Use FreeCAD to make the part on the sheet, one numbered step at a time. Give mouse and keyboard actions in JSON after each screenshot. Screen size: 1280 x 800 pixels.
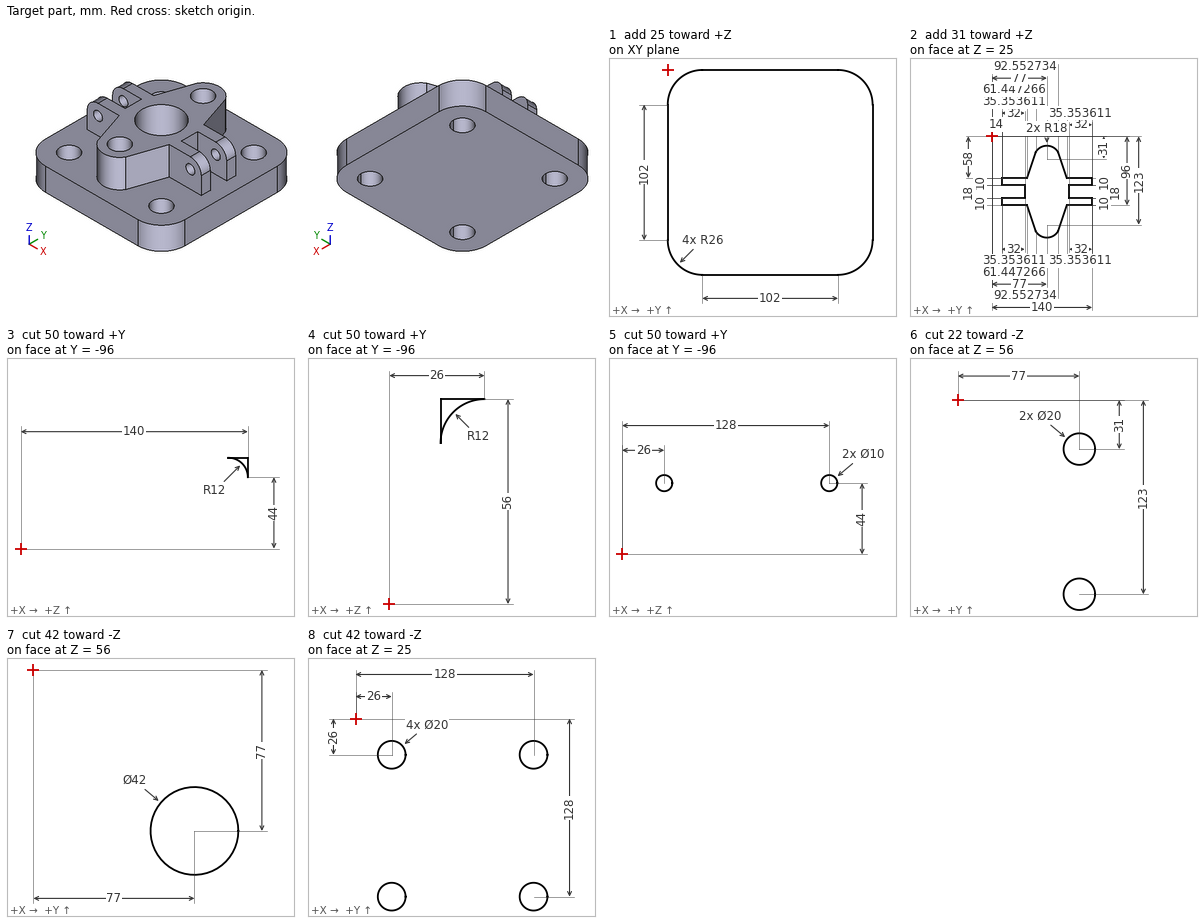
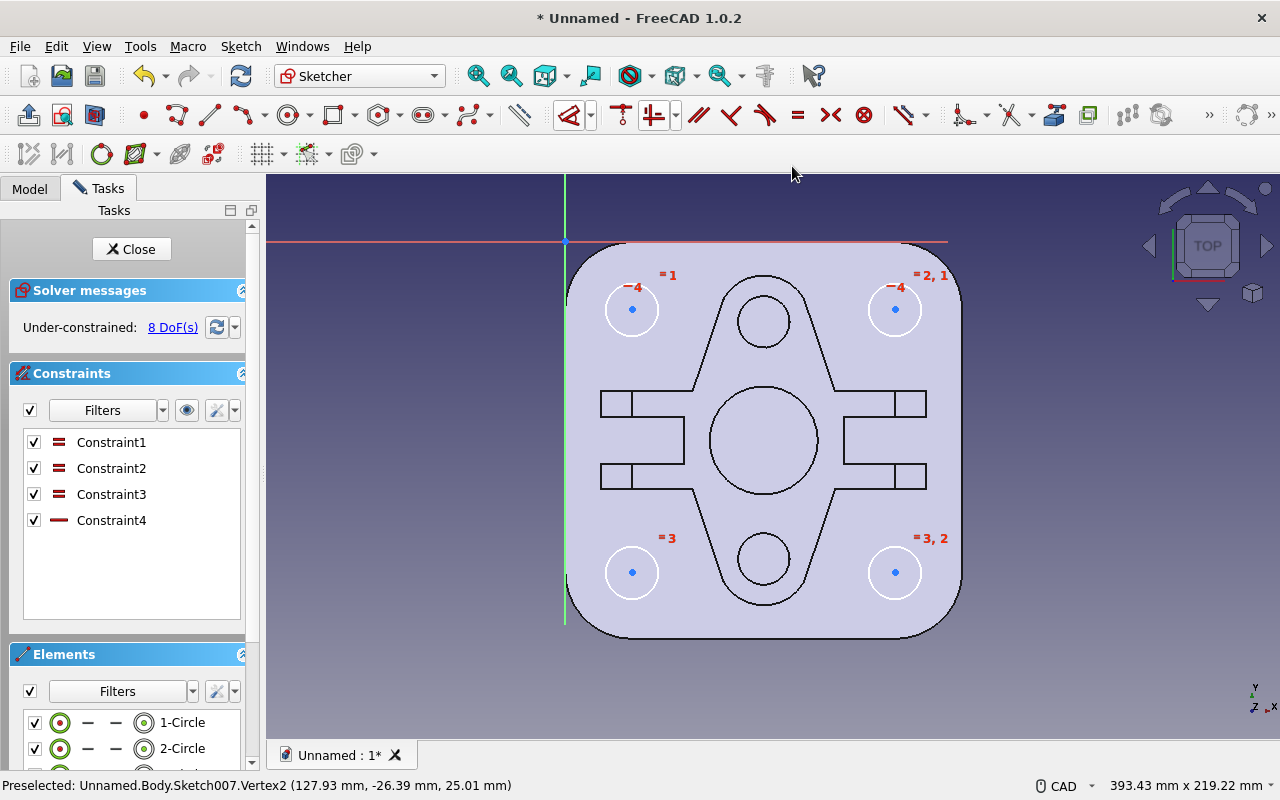
{"action": "left_click", "coordinate": [895, 310]}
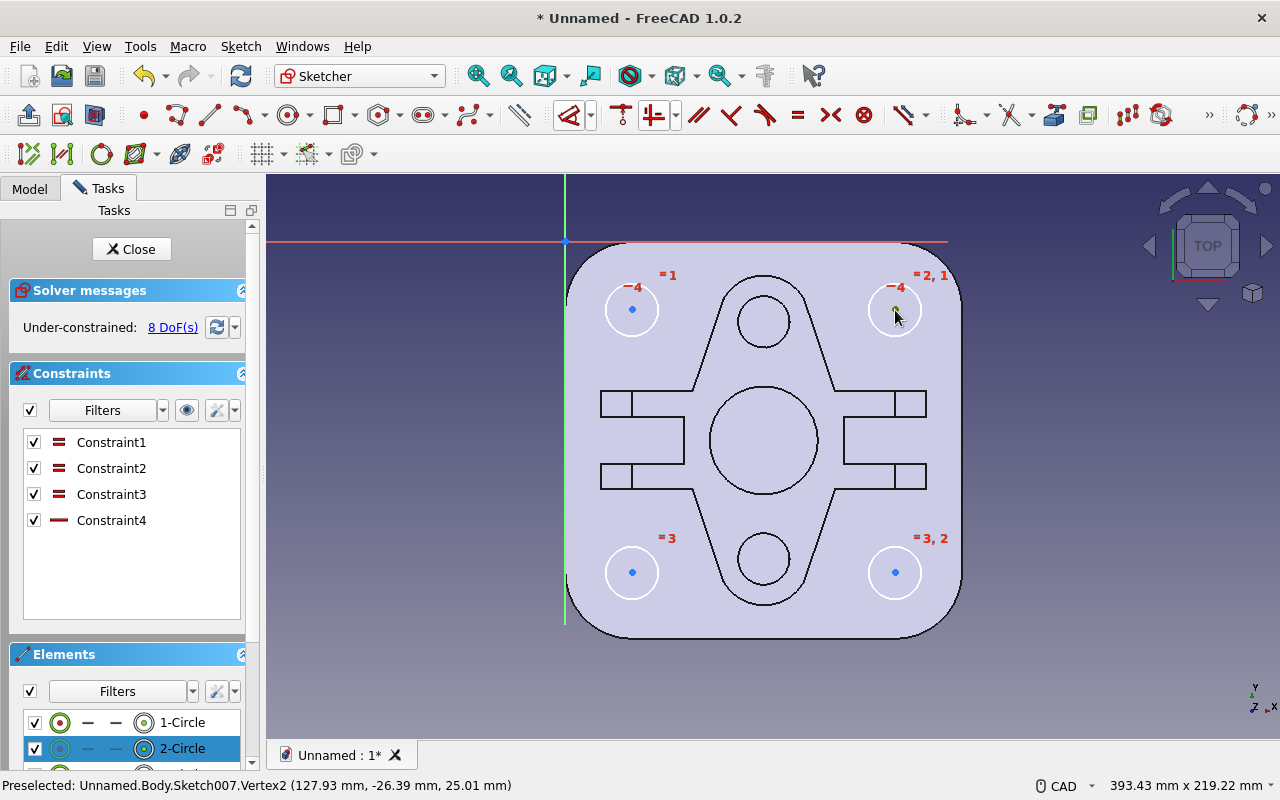
{"action": "left_click", "coordinate": [895, 573]}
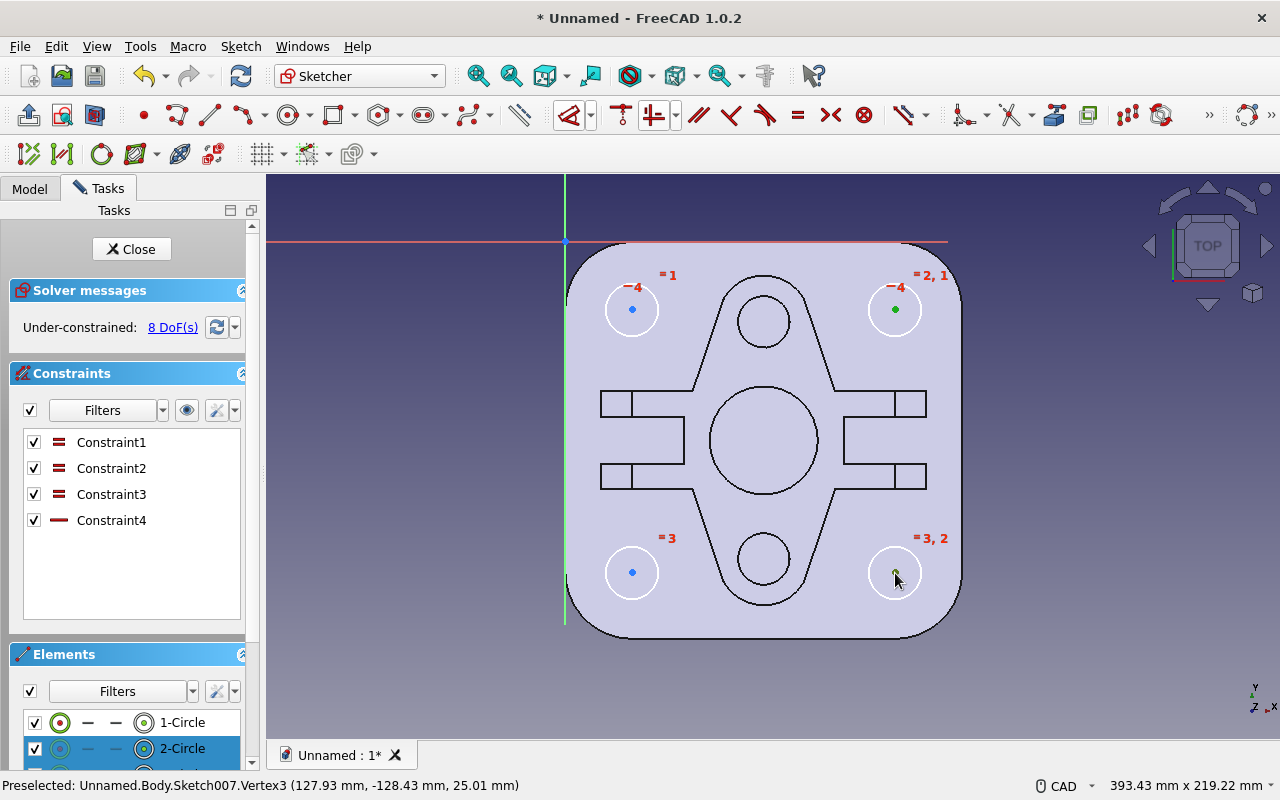
{"action": "key", "text": "v"}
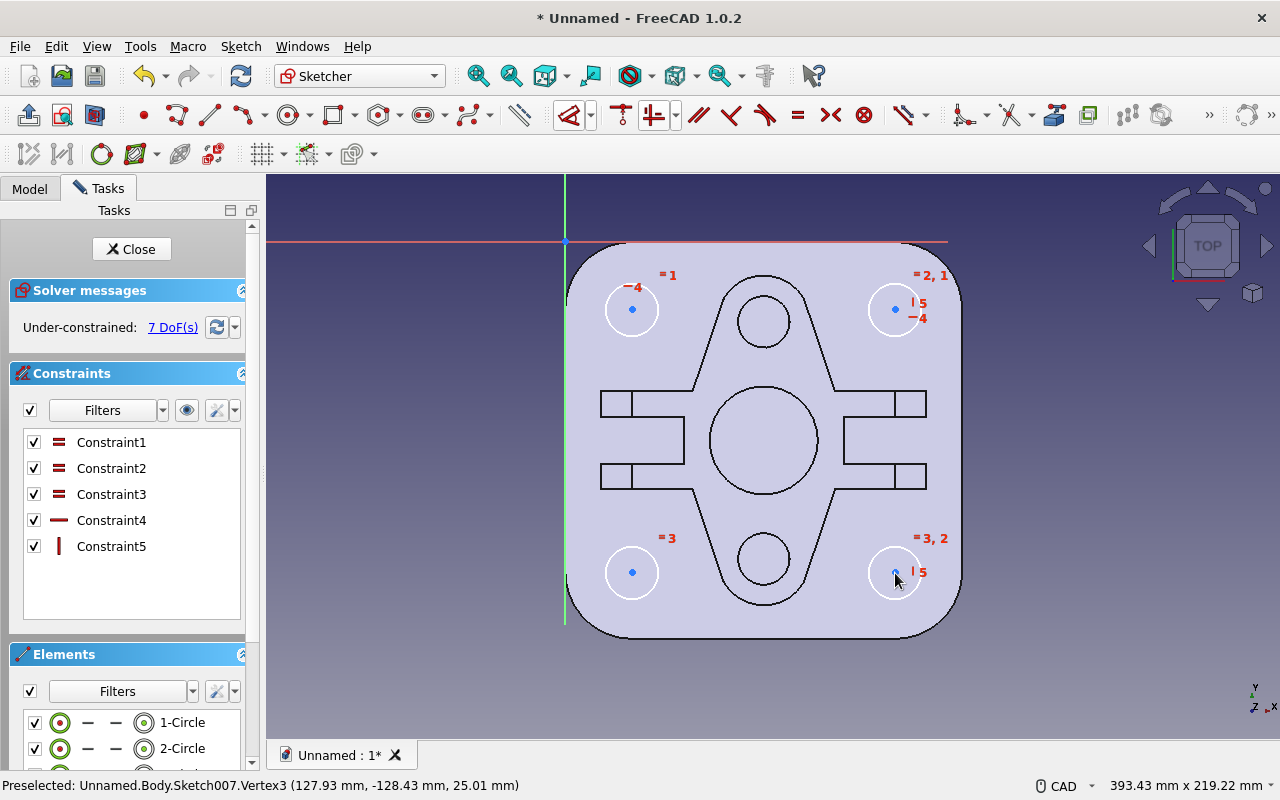
{"action": "left_click", "coordinate": [632, 310]}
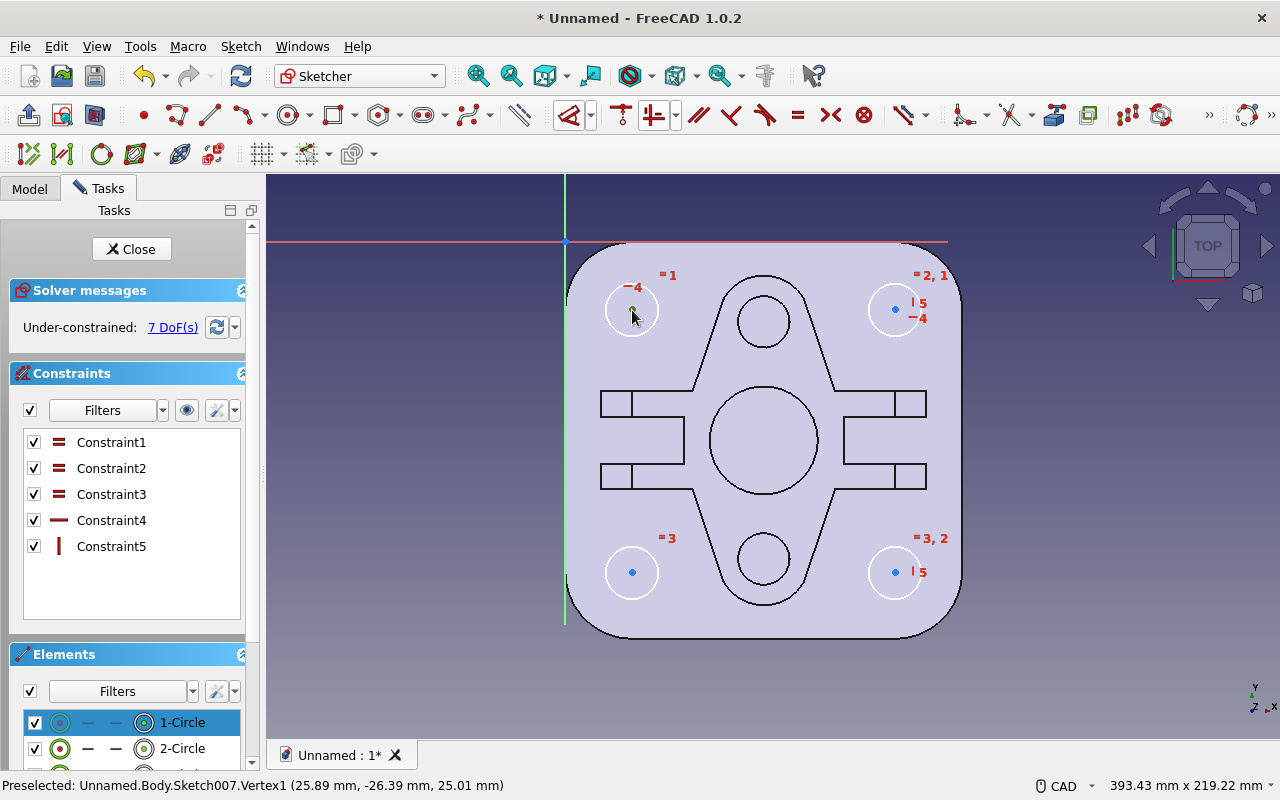
{"action": "left_click", "coordinate": [632, 573]}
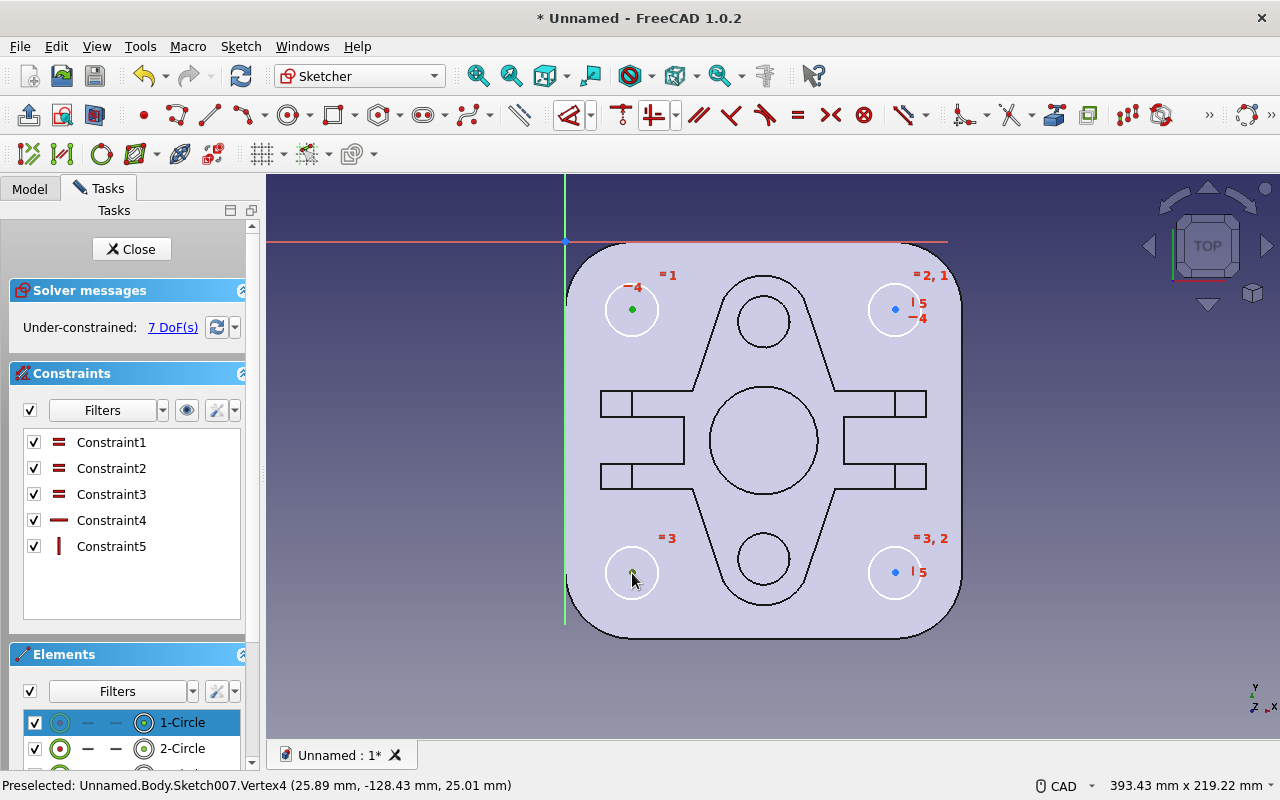
{"action": "left_click", "coordinate": [676, 116]}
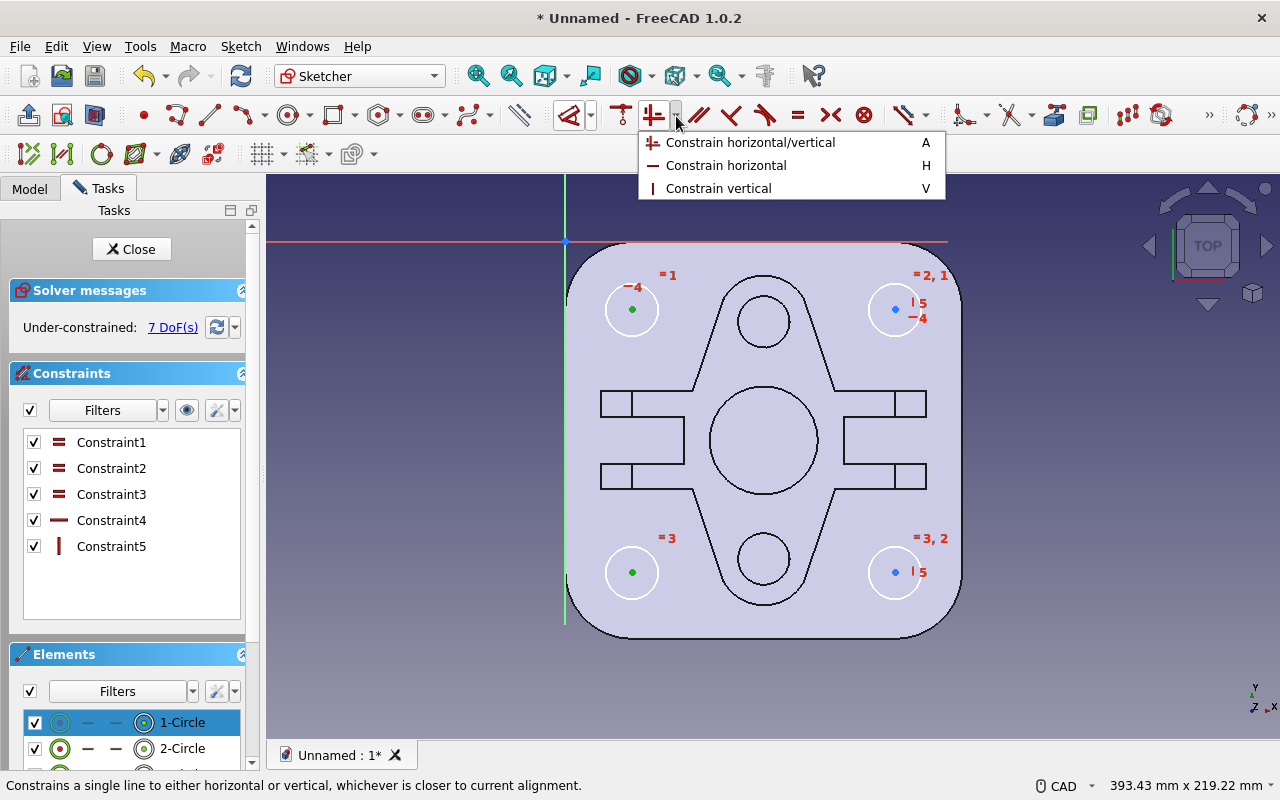
{"action": "left_click", "coordinate": [792, 188]}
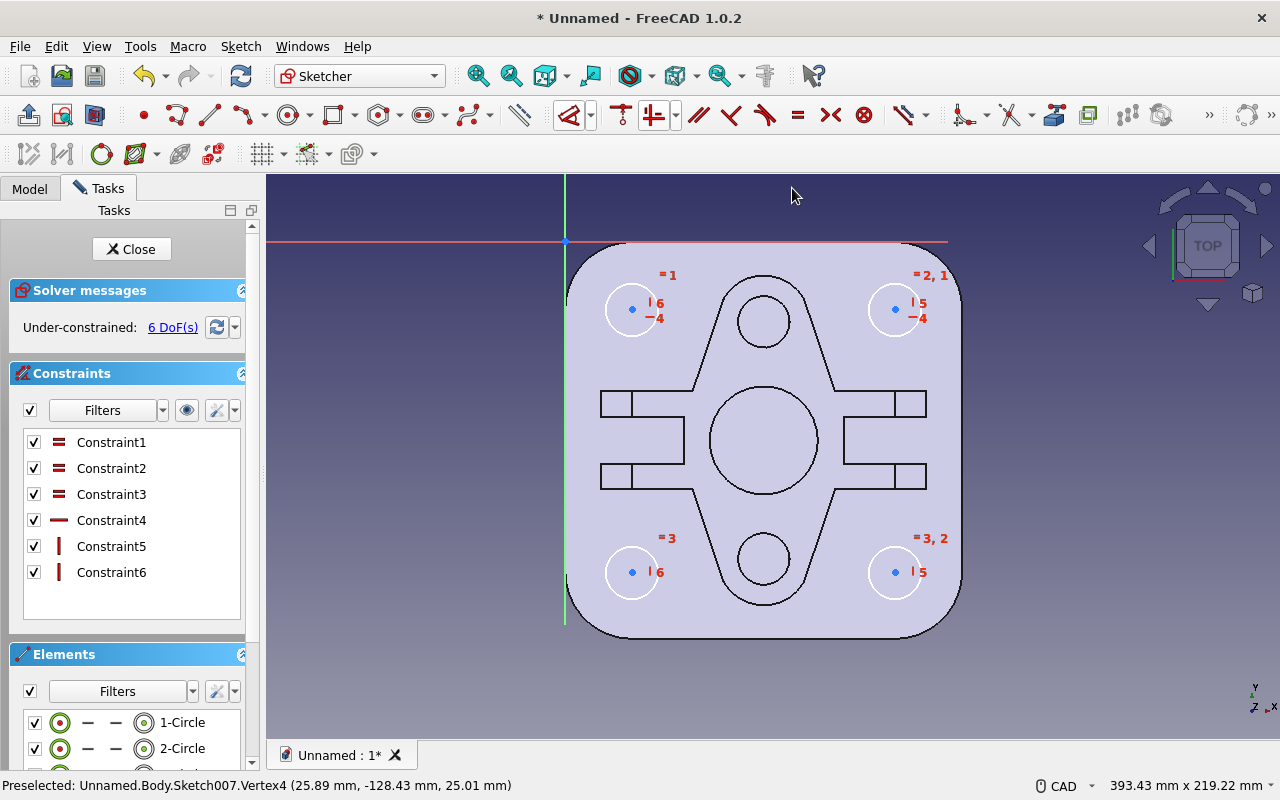
{"action": "left_click", "coordinate": [895, 573]}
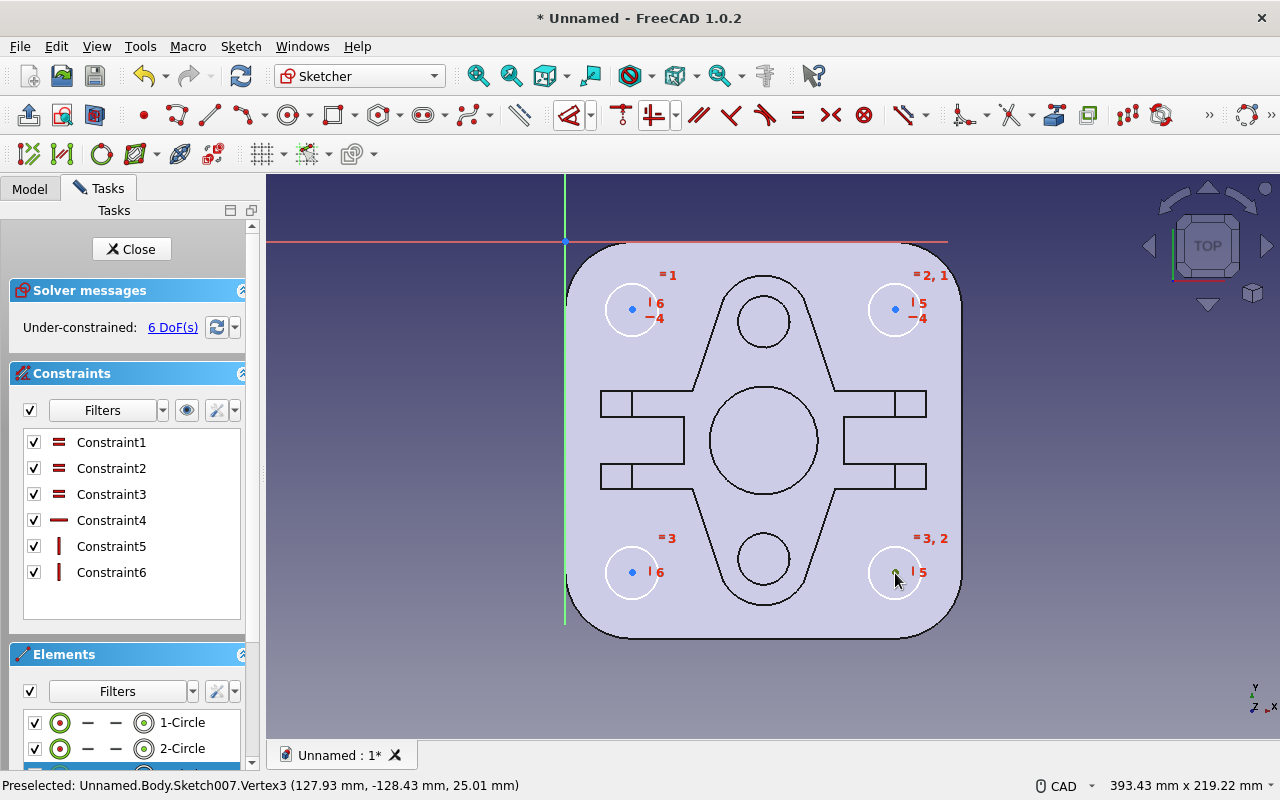
{"action": "left_click", "coordinate": [632, 573]}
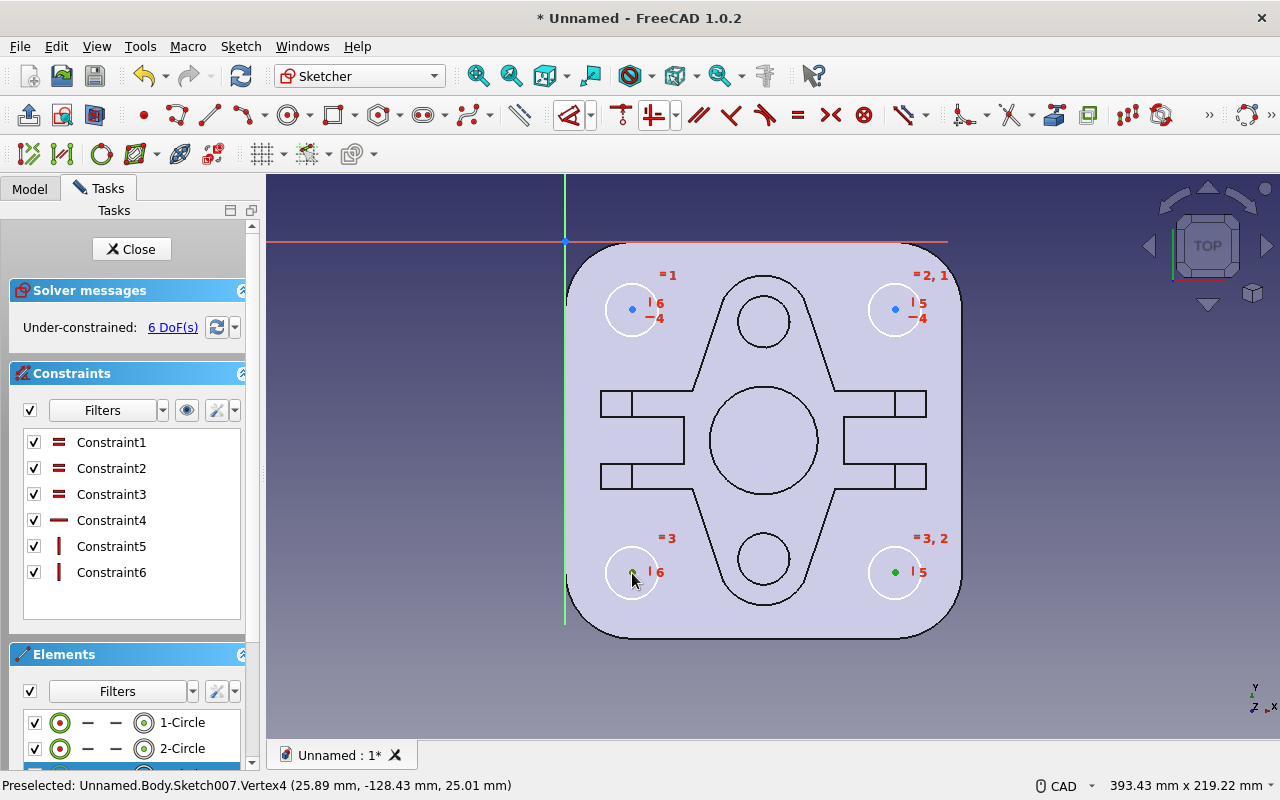
{"action": "left_click", "coordinate": [676, 116]}